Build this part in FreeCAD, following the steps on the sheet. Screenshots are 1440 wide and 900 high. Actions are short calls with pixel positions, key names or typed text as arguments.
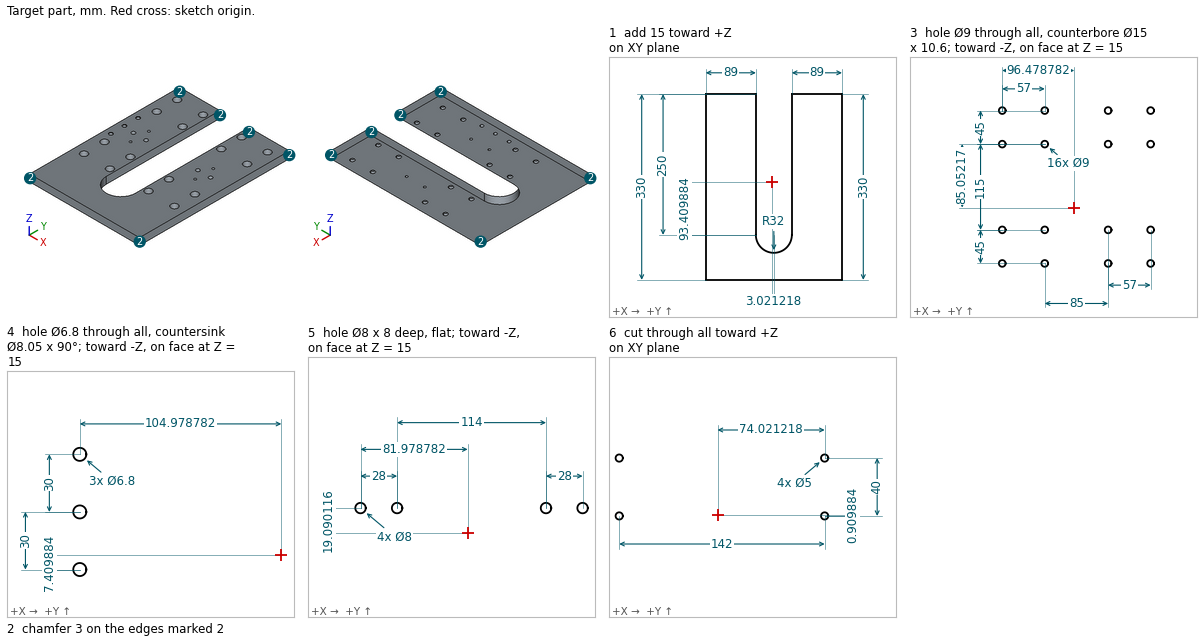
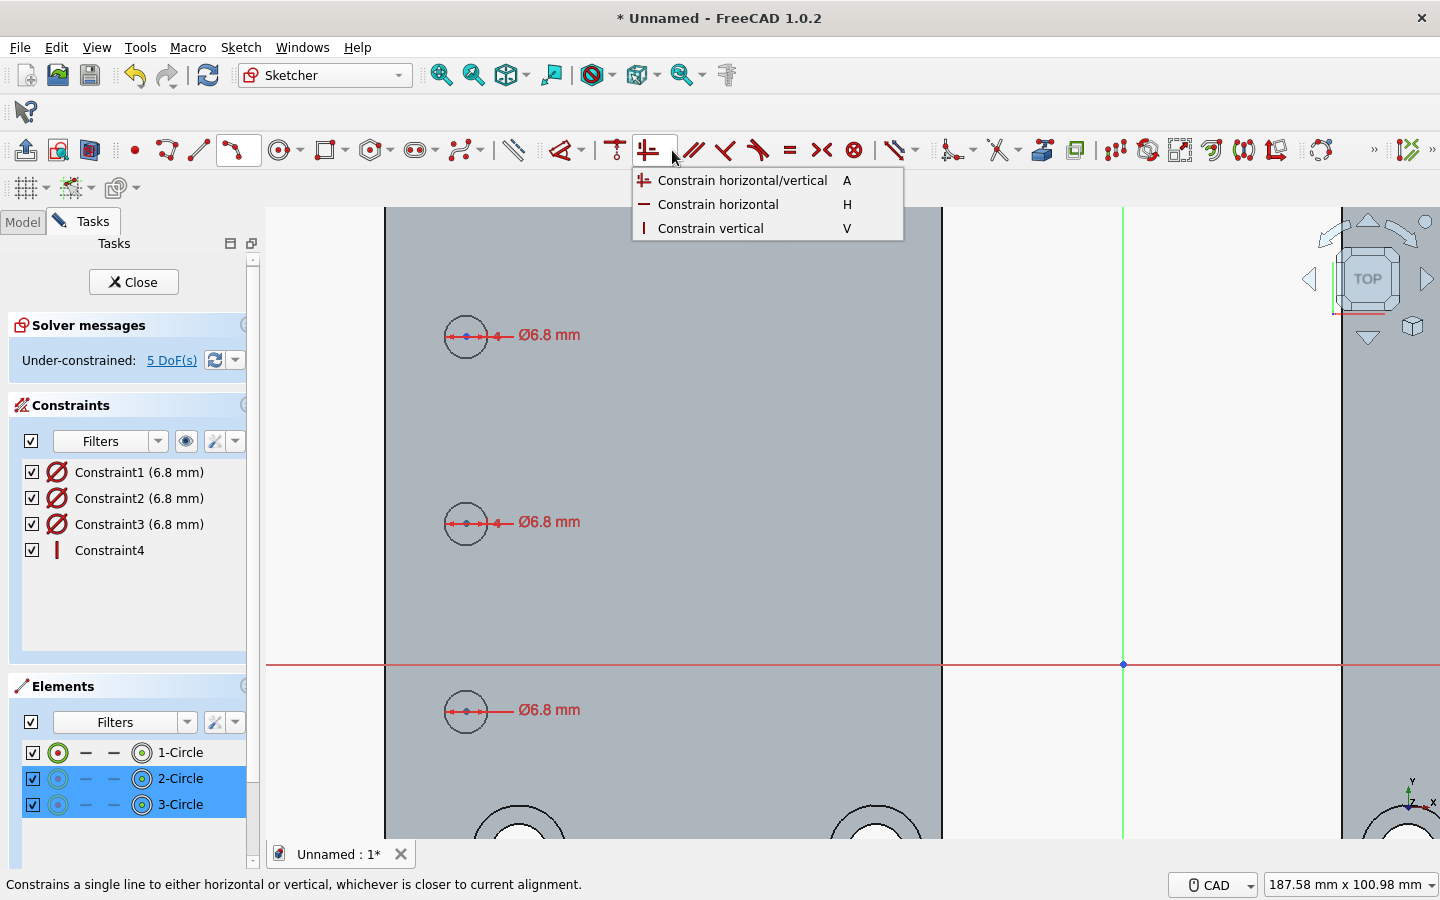
click(768, 228)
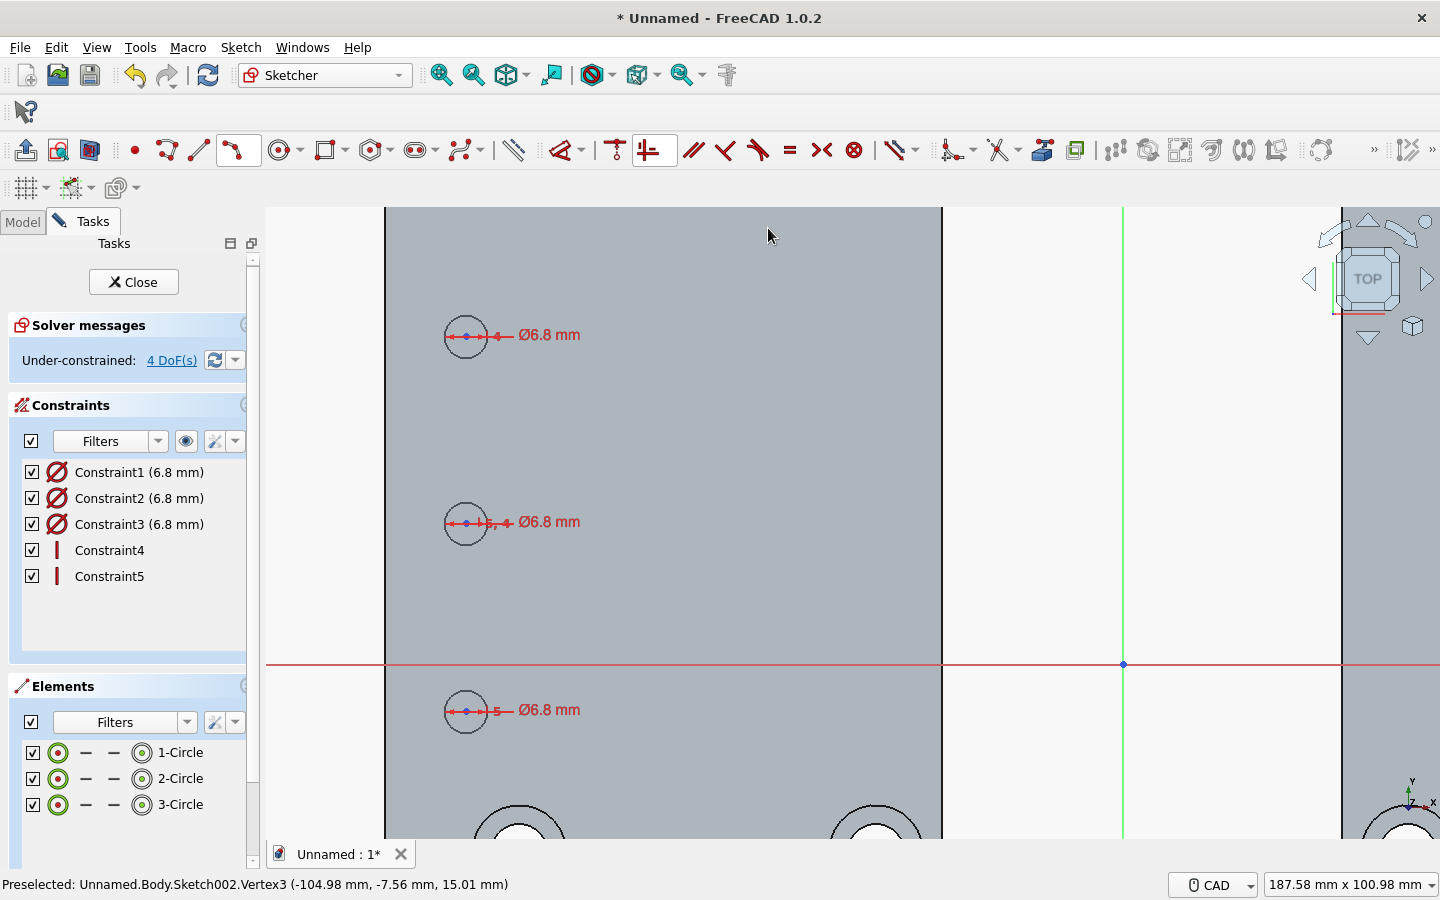
click(560, 150)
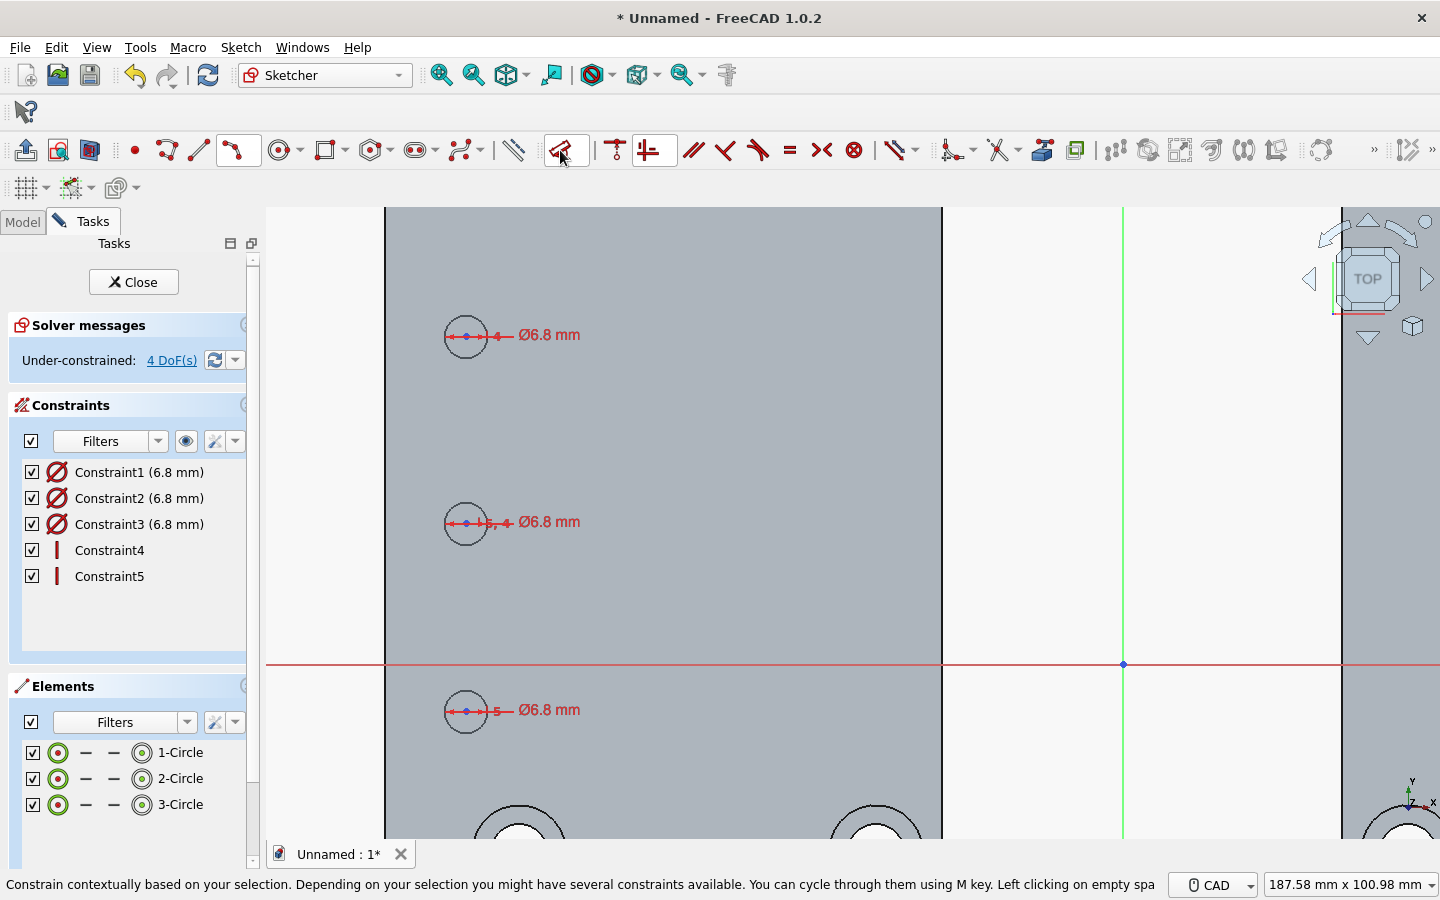
click(466, 337)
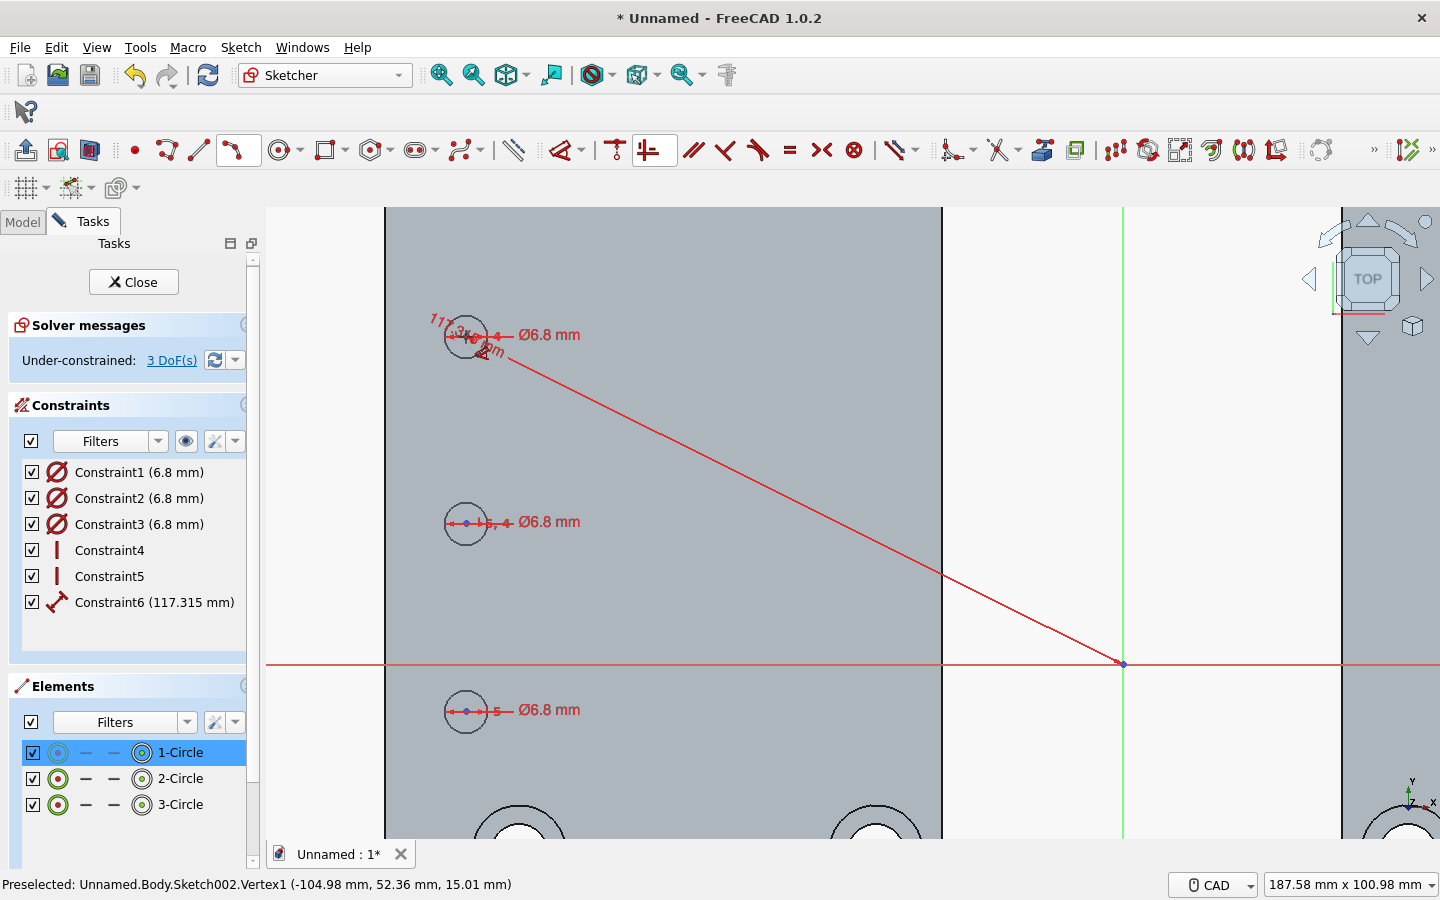
click(466, 524)
click(432, 431)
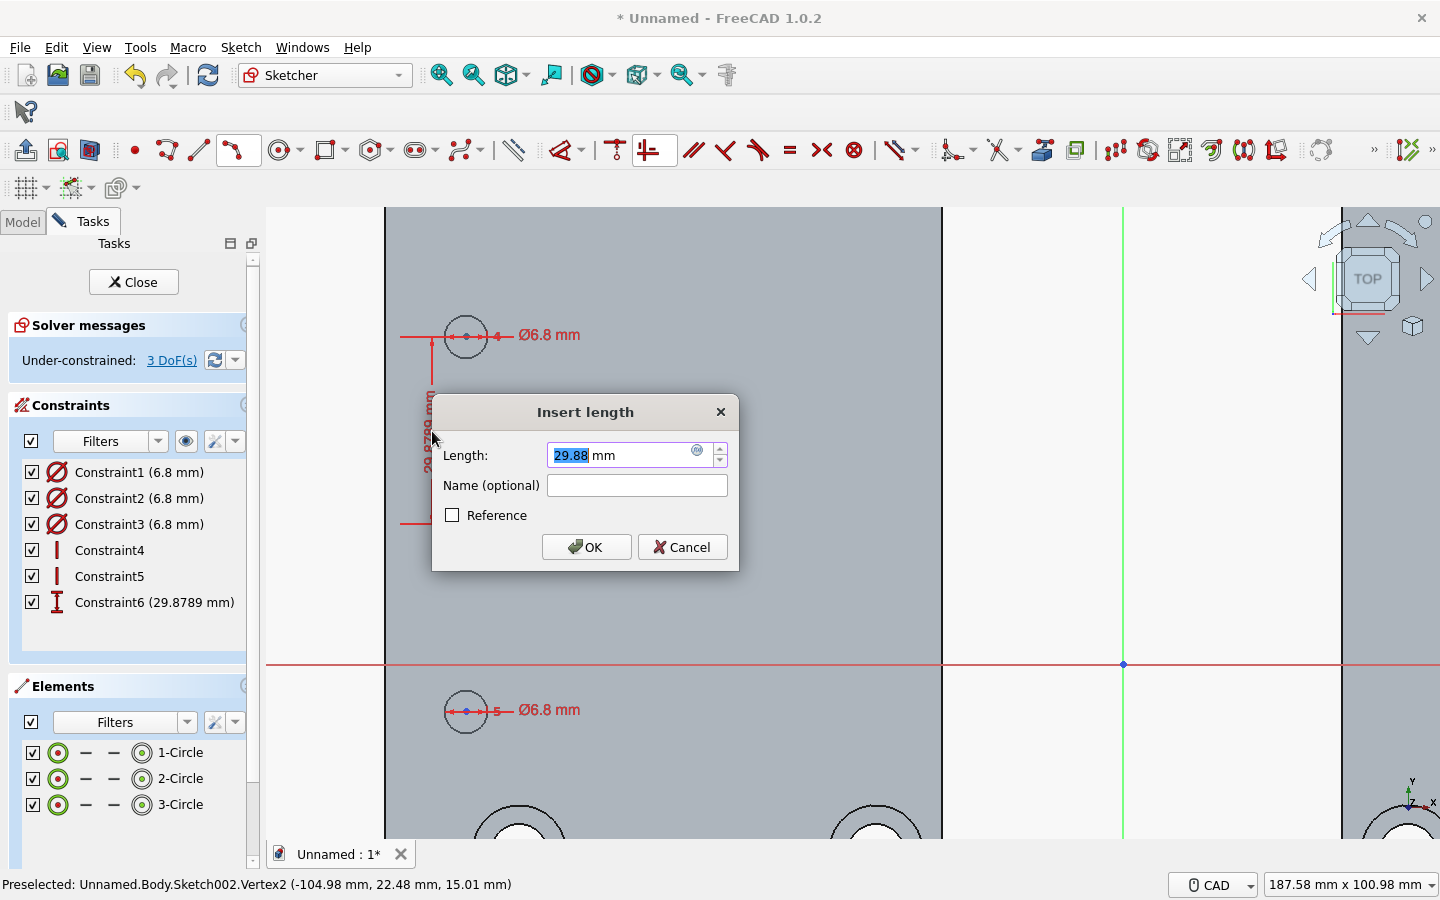
text(30)
key(Return)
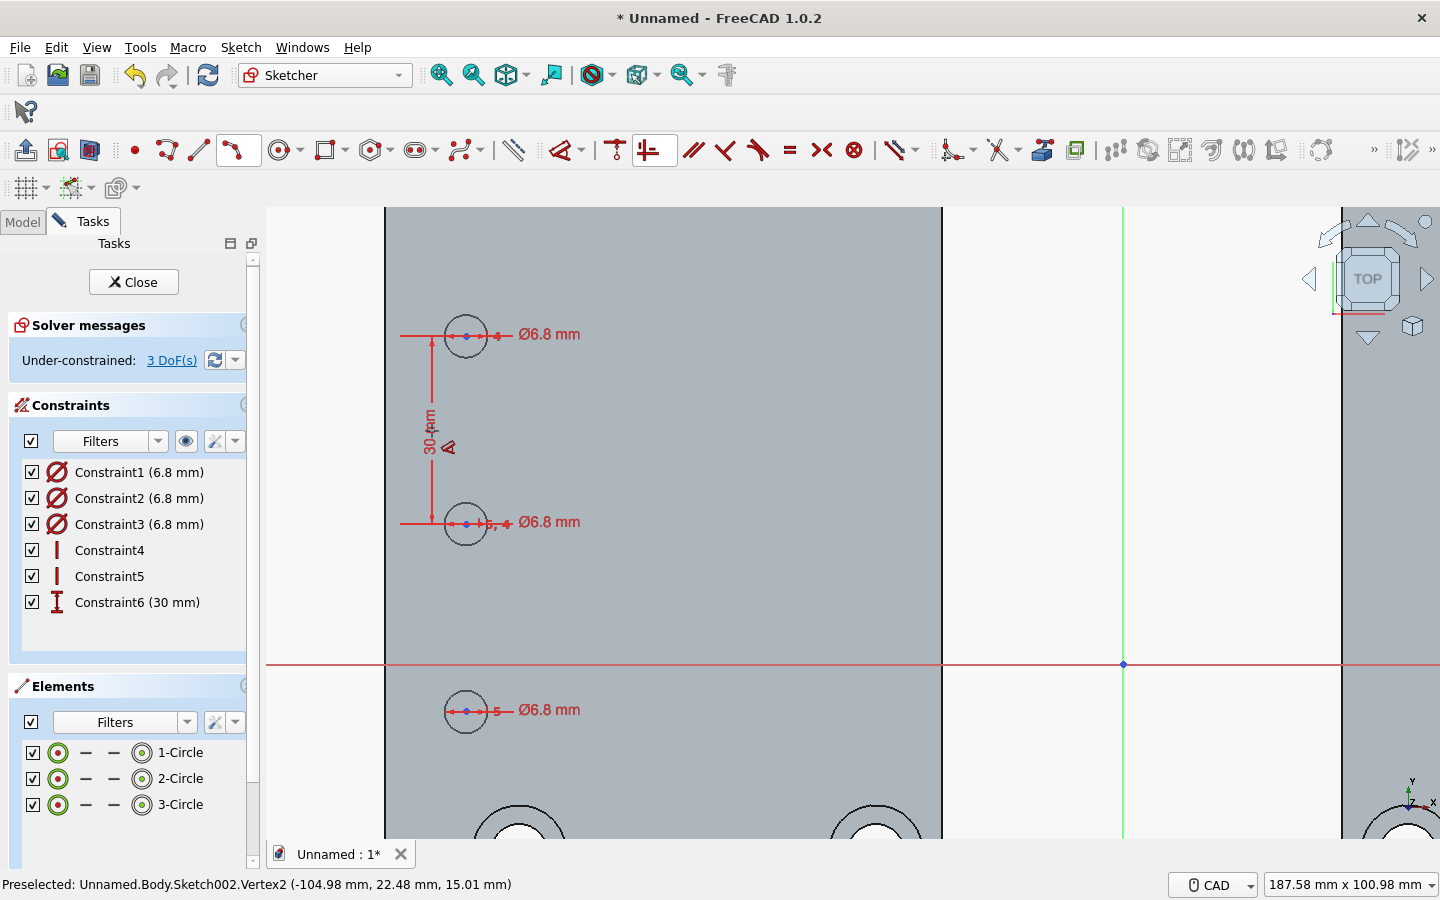
click(466, 524)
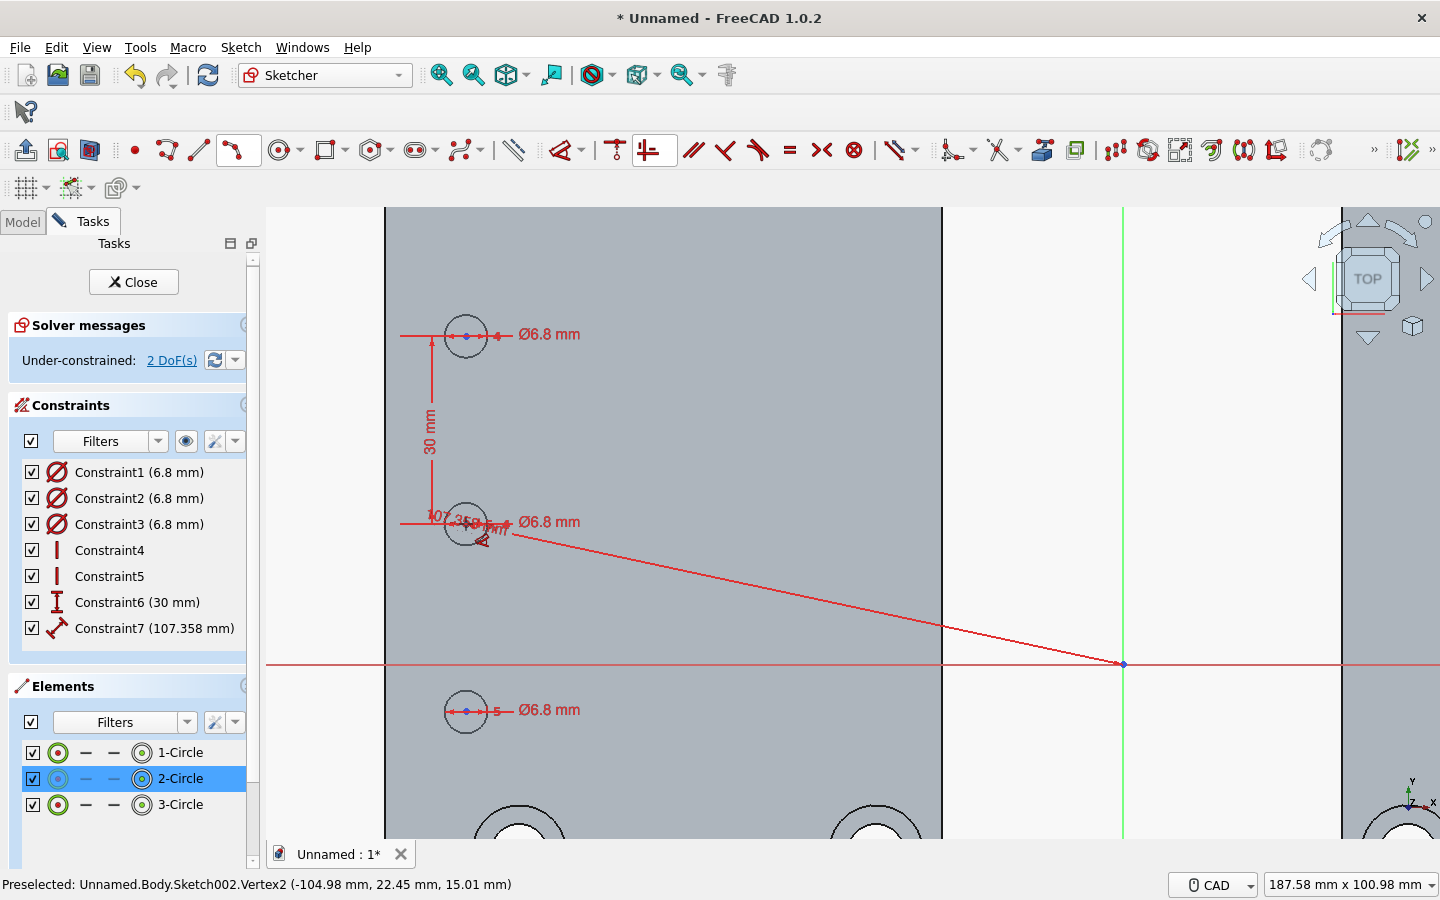
click(466, 712)
click(432, 618)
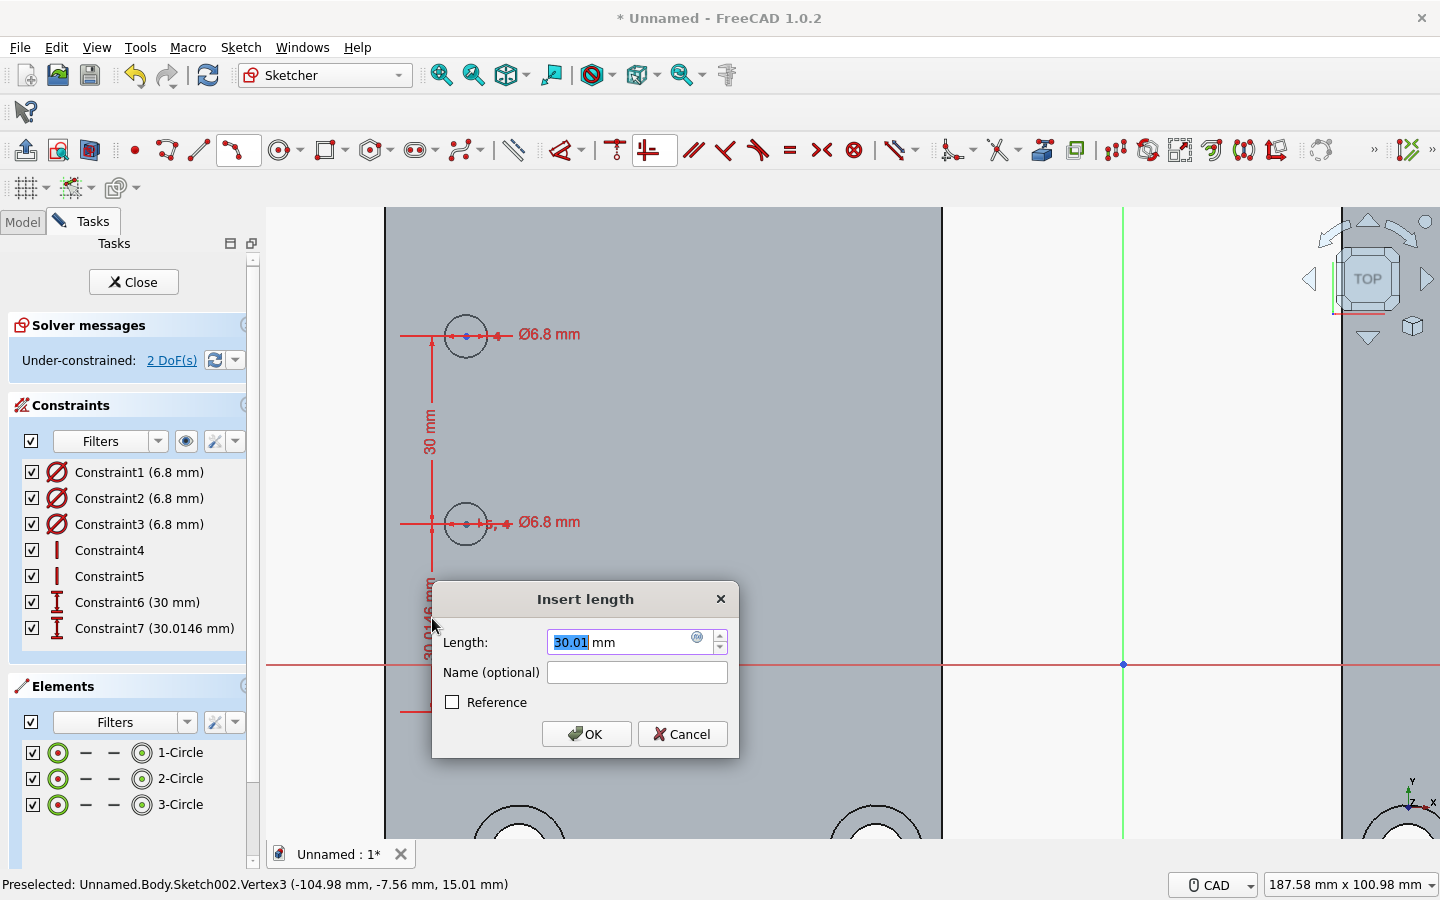
text(30)
key(Return)